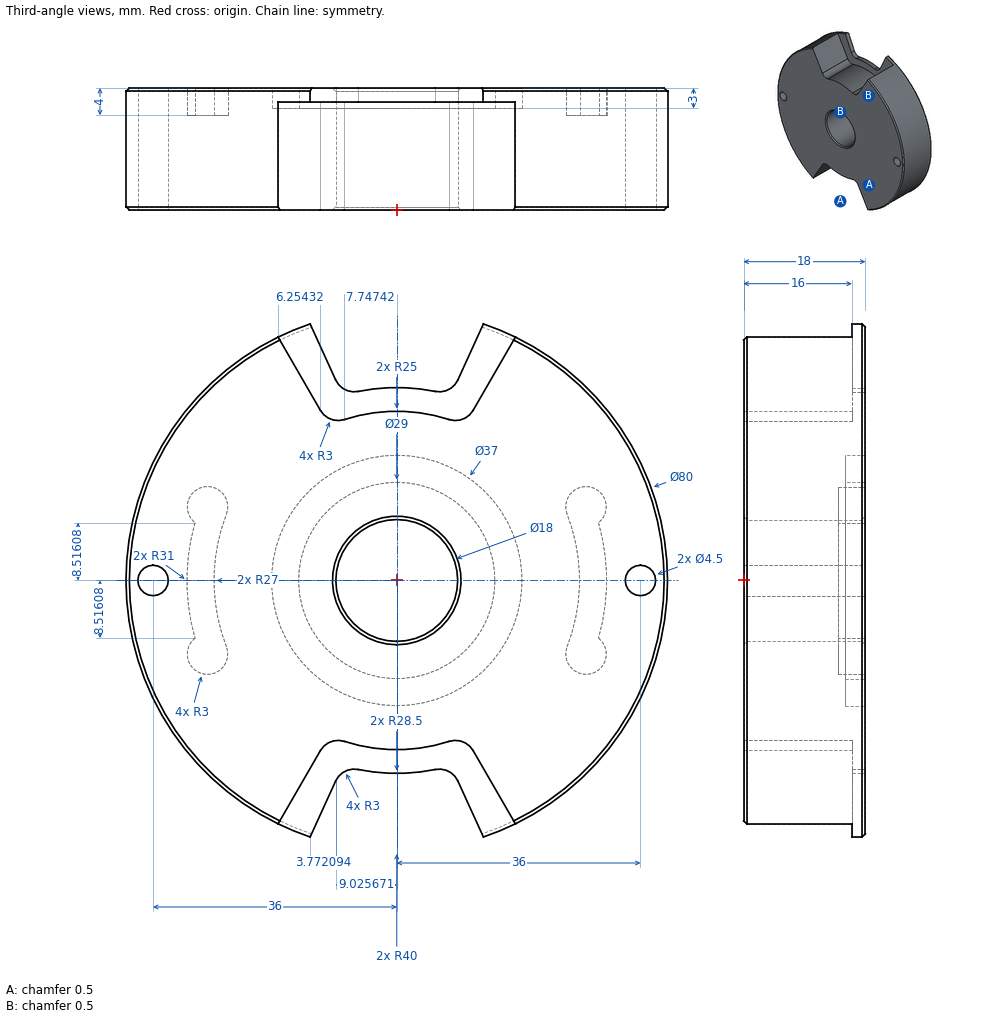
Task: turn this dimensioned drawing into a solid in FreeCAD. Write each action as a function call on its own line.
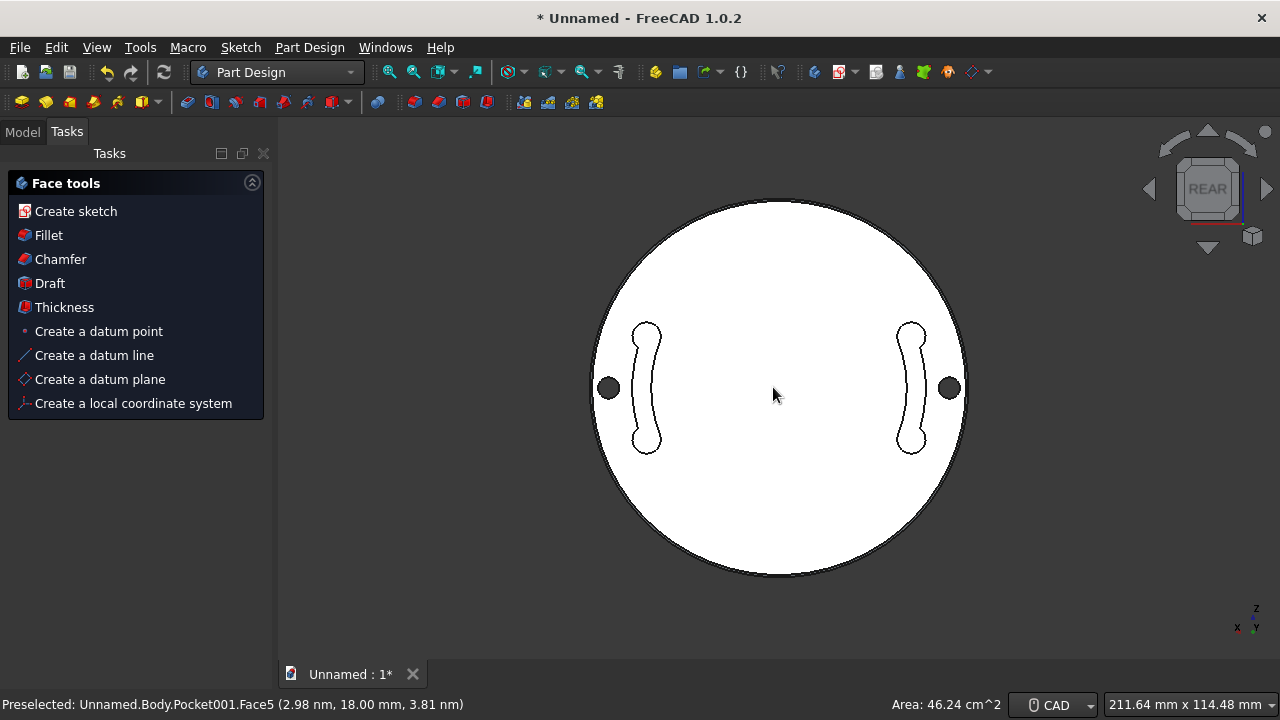
click(840, 72)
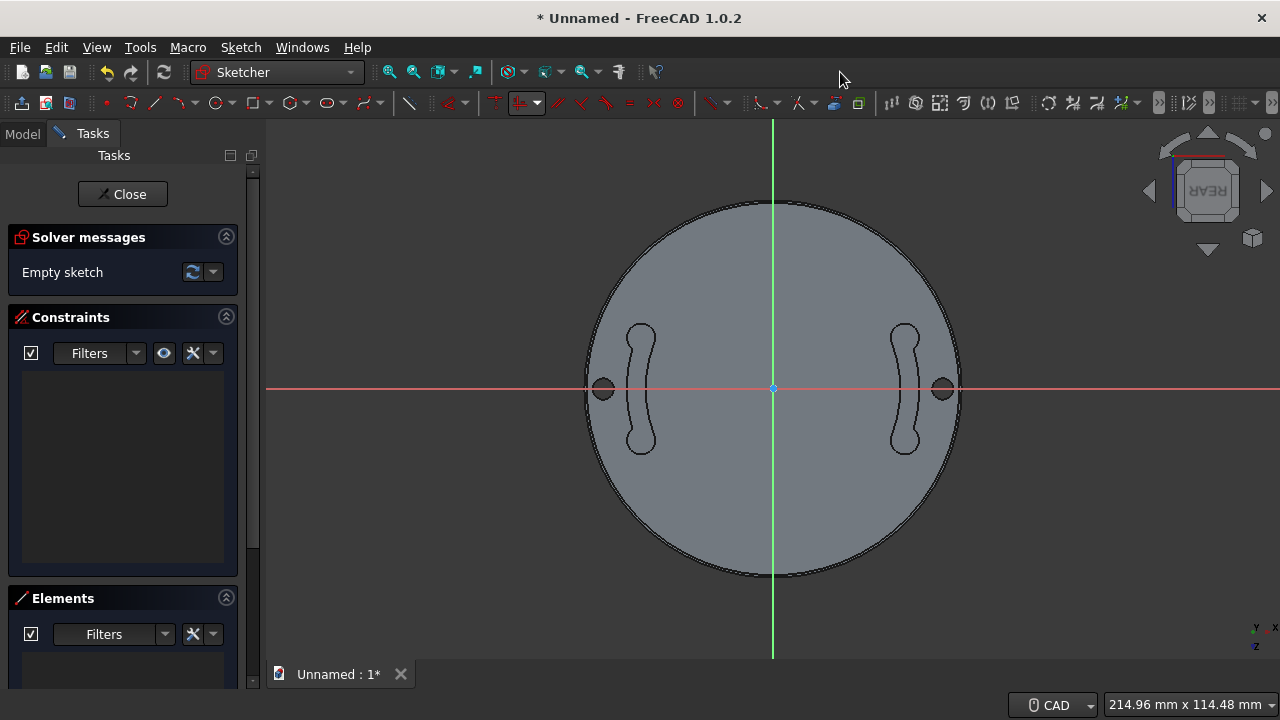
click(156, 104)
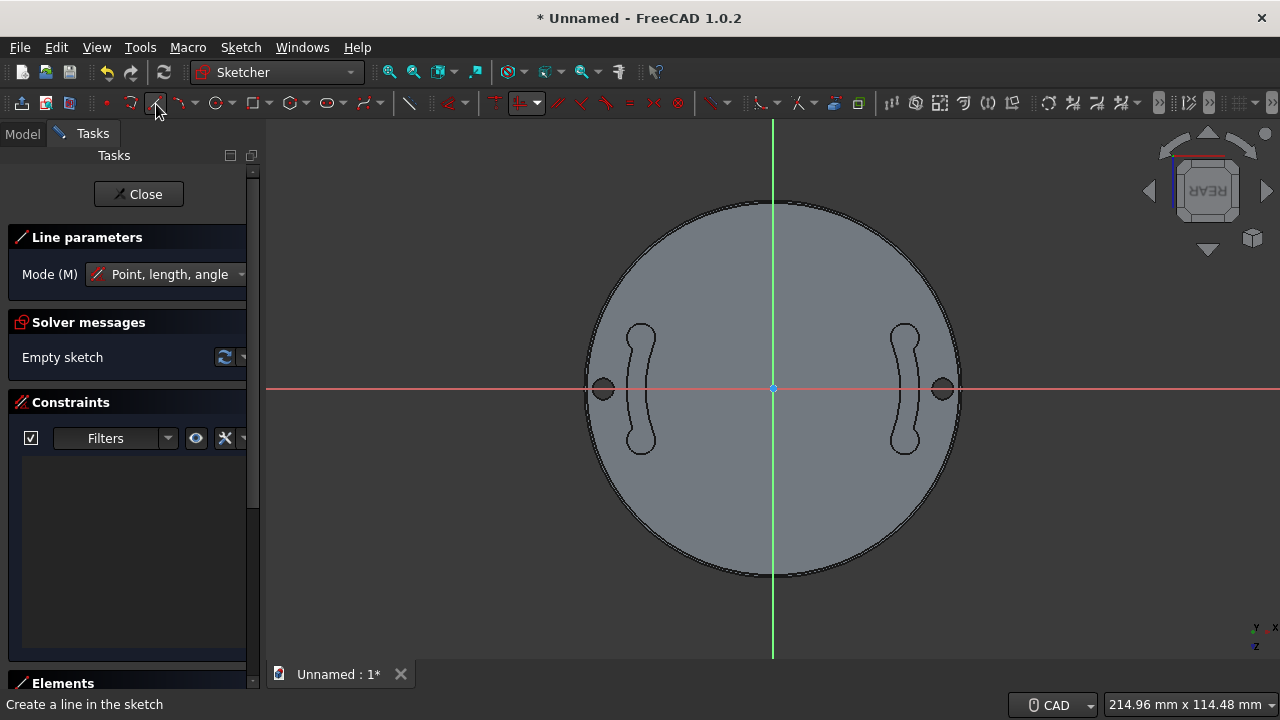
click(713, 210)
click(730, 249)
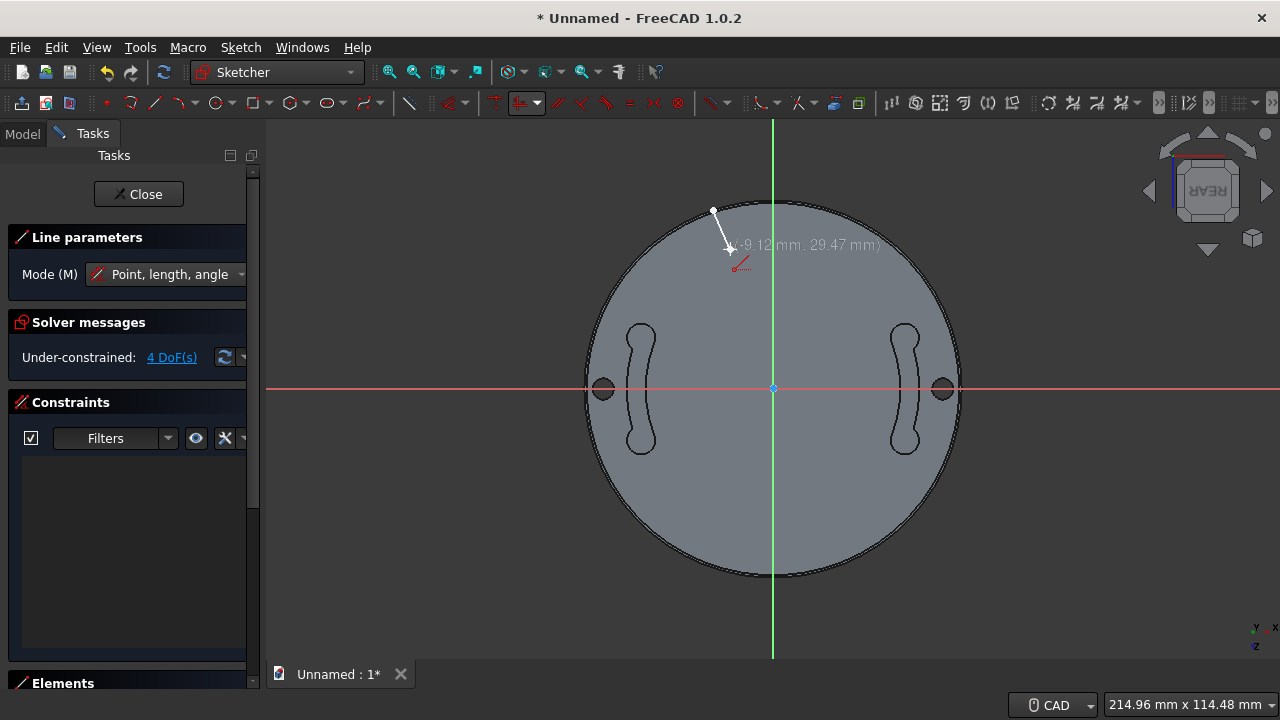
click(816, 249)
click(833, 210)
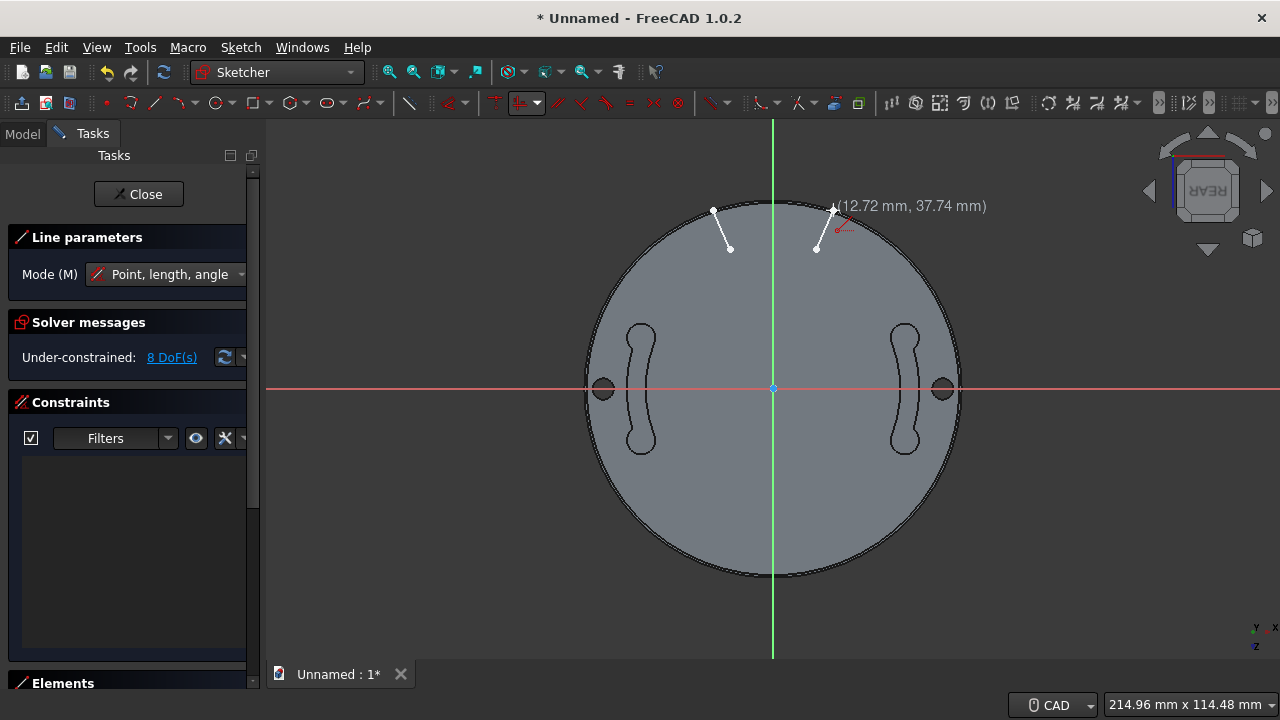
click(180, 104)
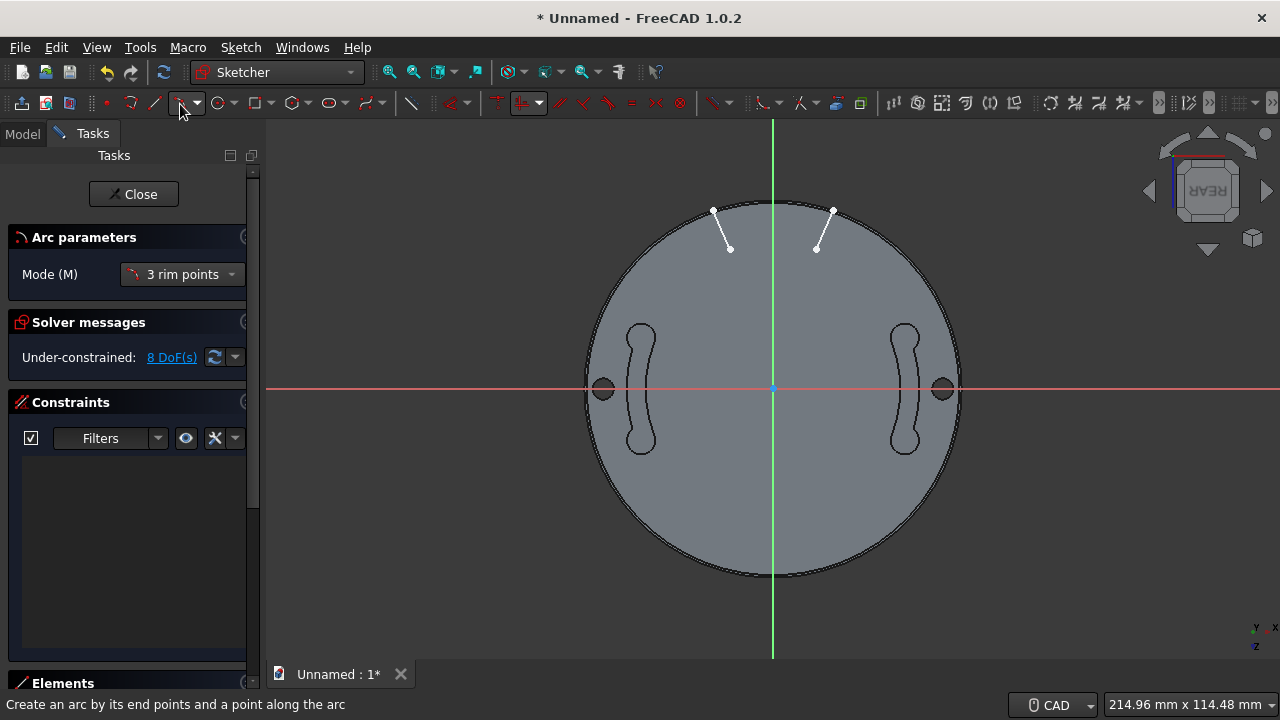
click(730, 250)
click(746, 257)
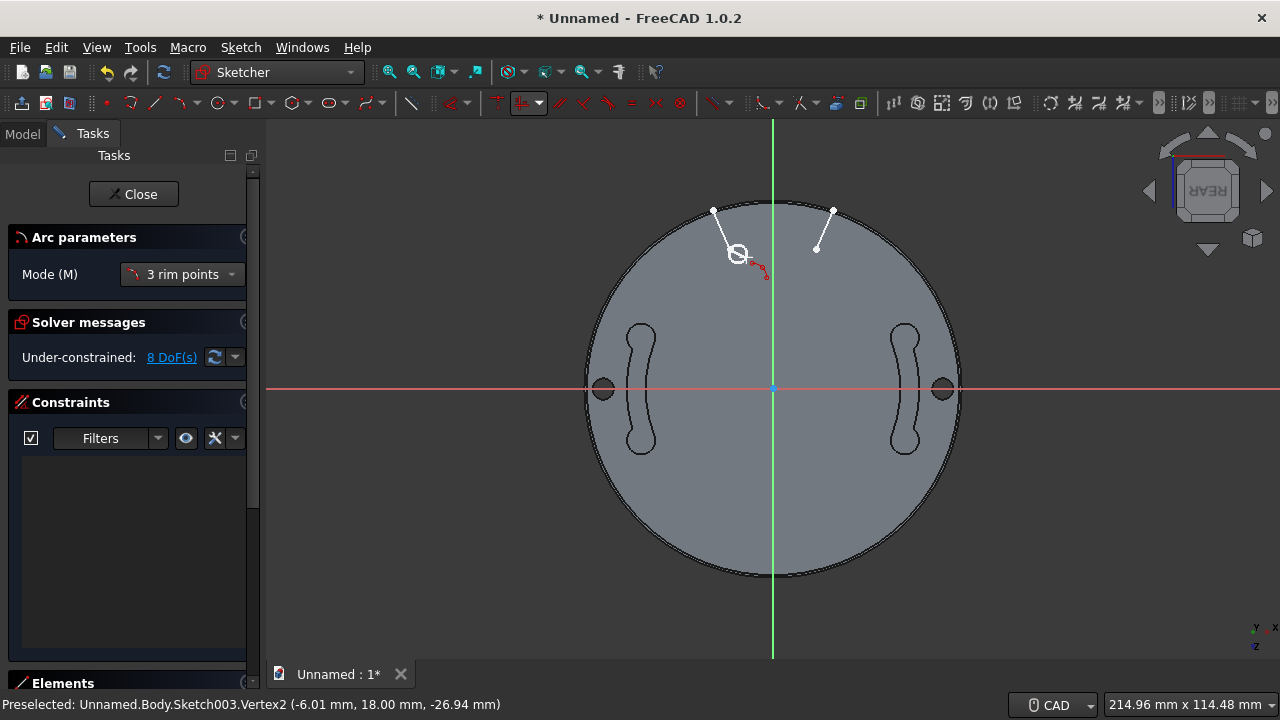
scroll(737, 256, up, 9)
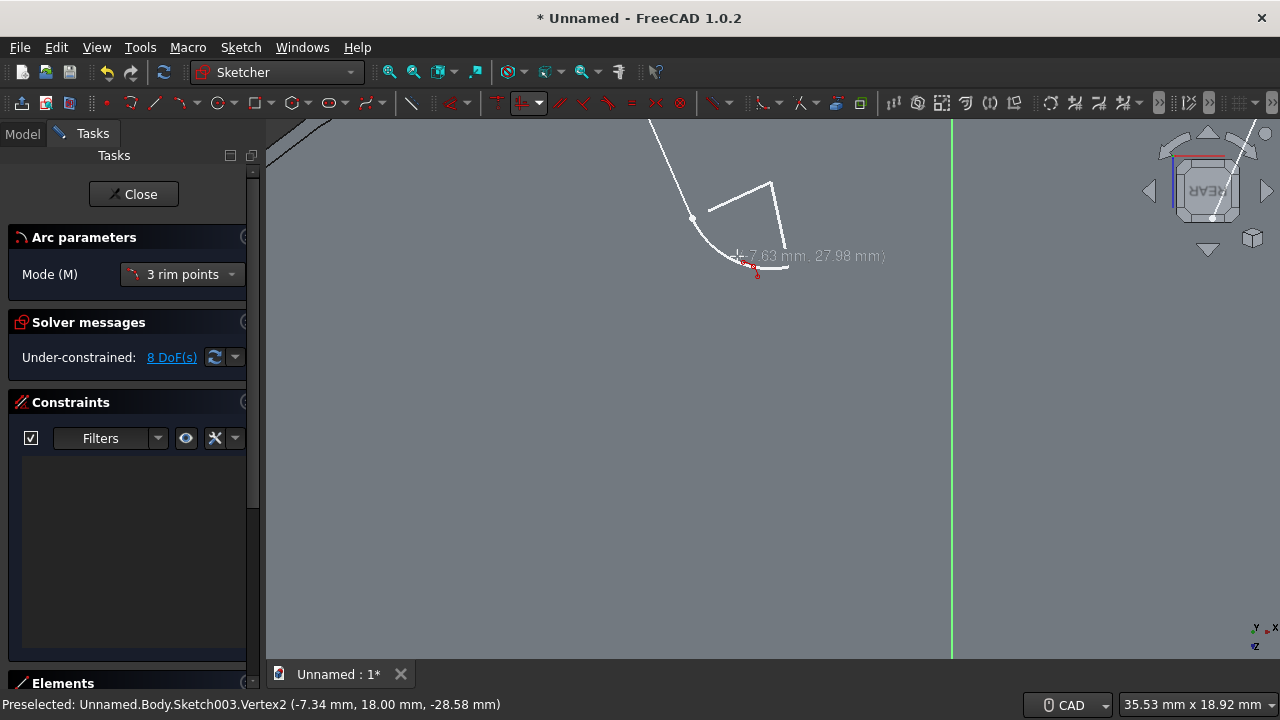
click(734, 255)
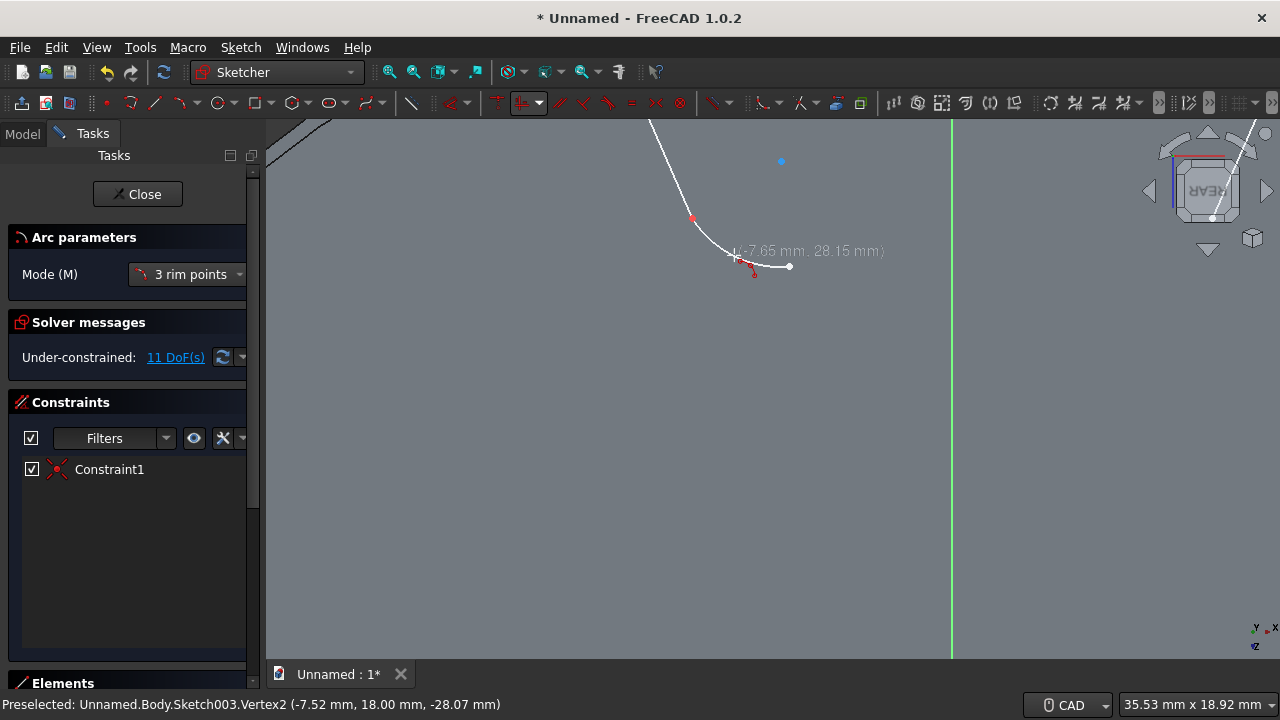
scroll(655, 256, down, 9)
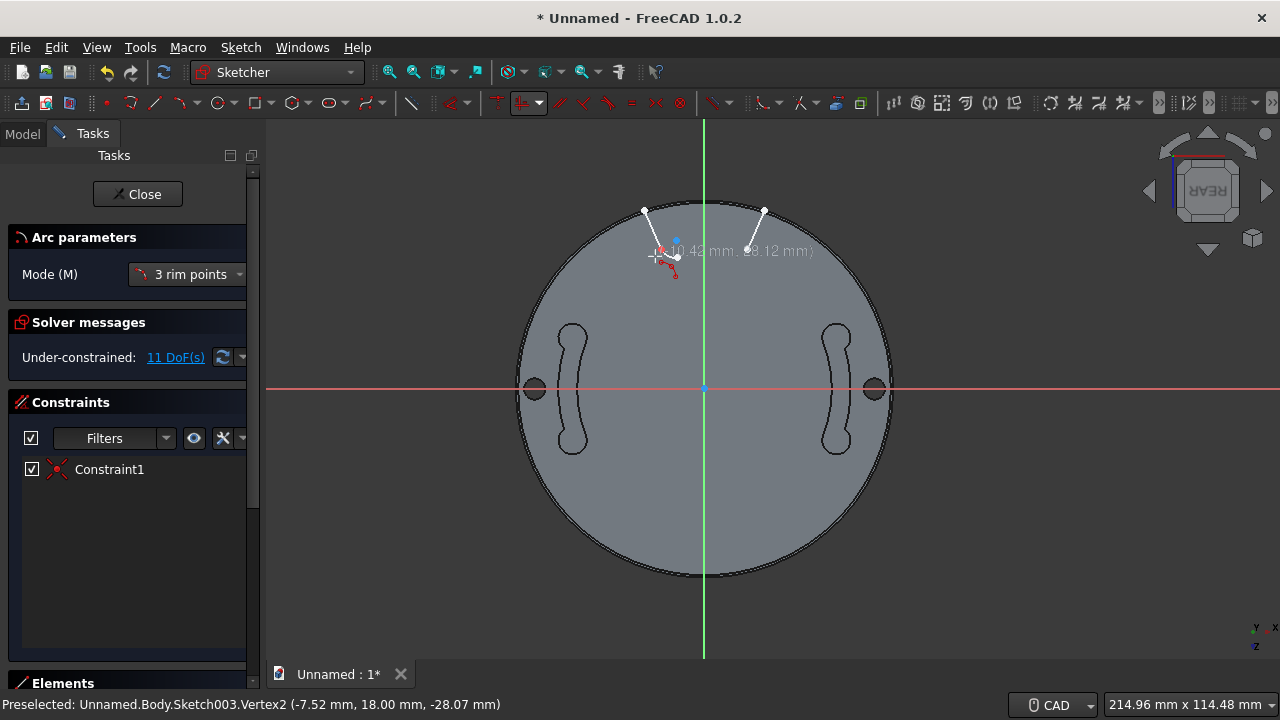
click(677, 258)
click(731, 257)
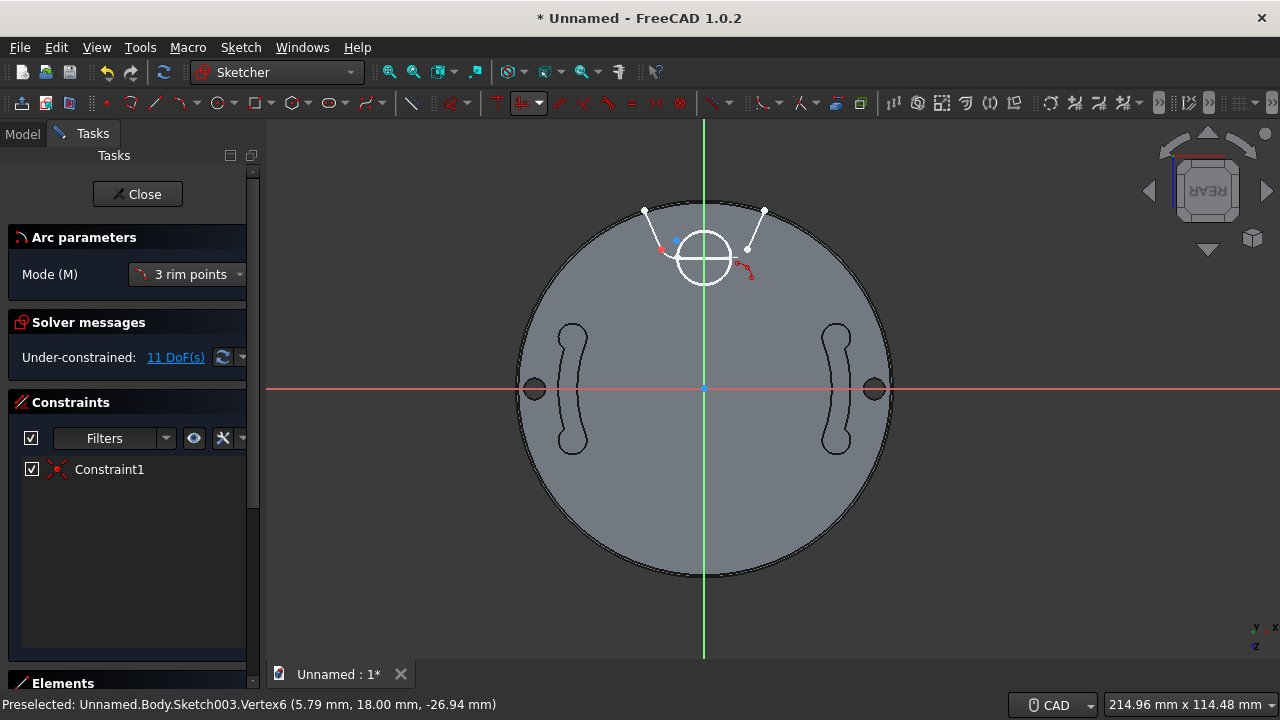
scroll(710, 255, up, 10)